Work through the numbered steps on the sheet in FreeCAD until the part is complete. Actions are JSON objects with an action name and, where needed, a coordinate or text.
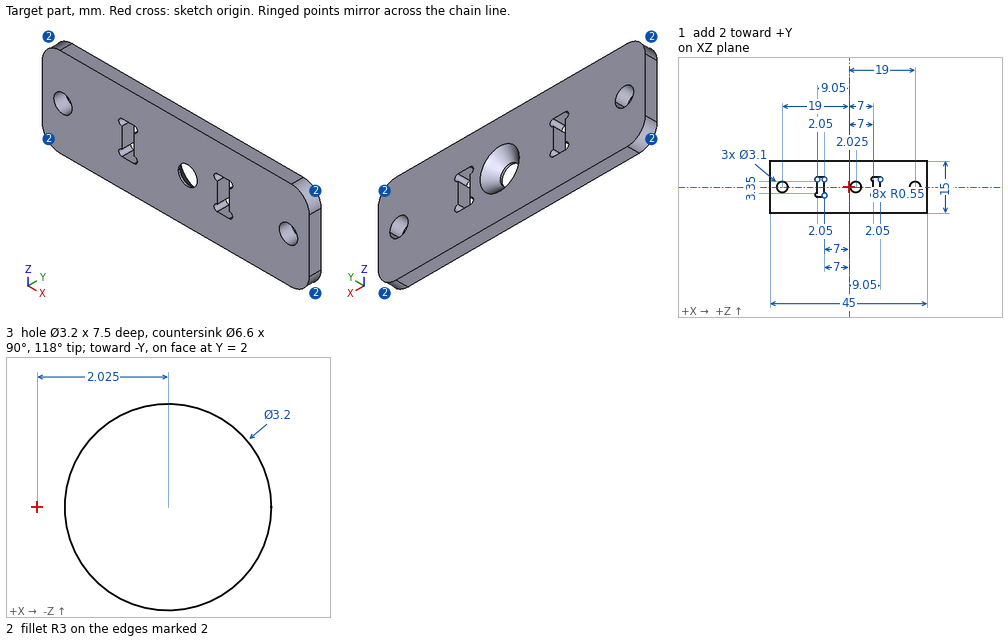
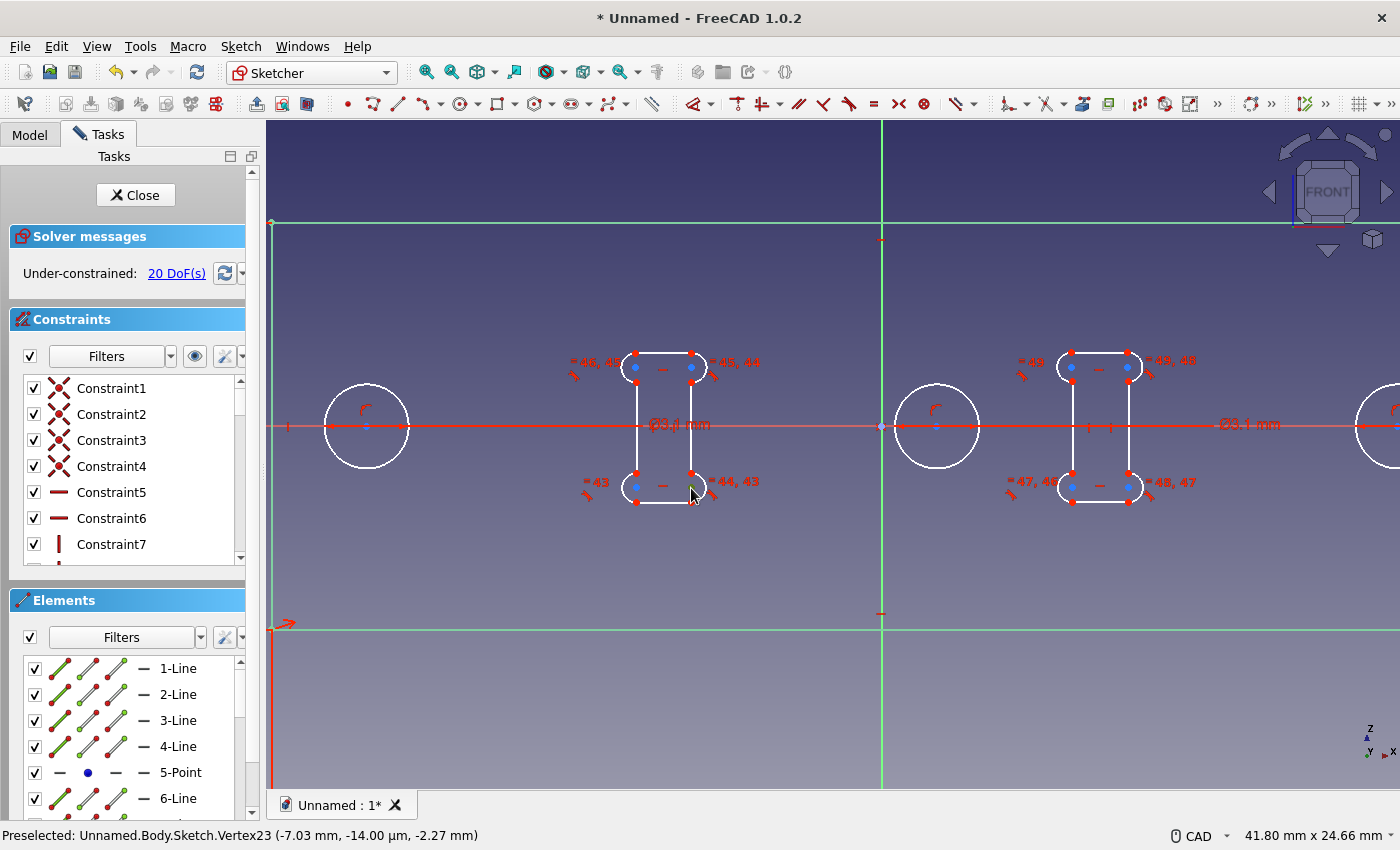
{"action": "left_click", "coordinate": [692, 368]}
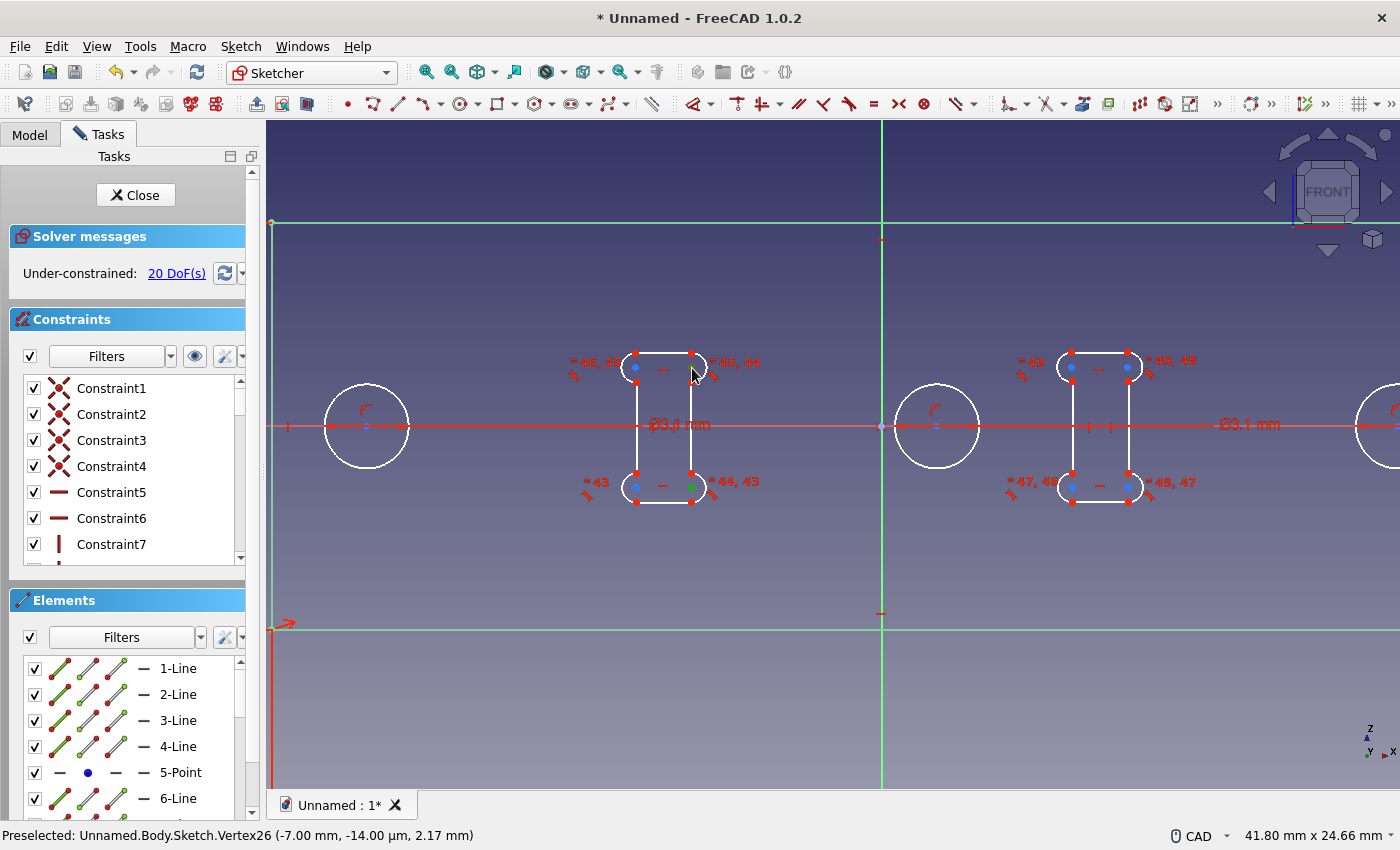
{"action": "left_click", "coordinate": [361, 426]}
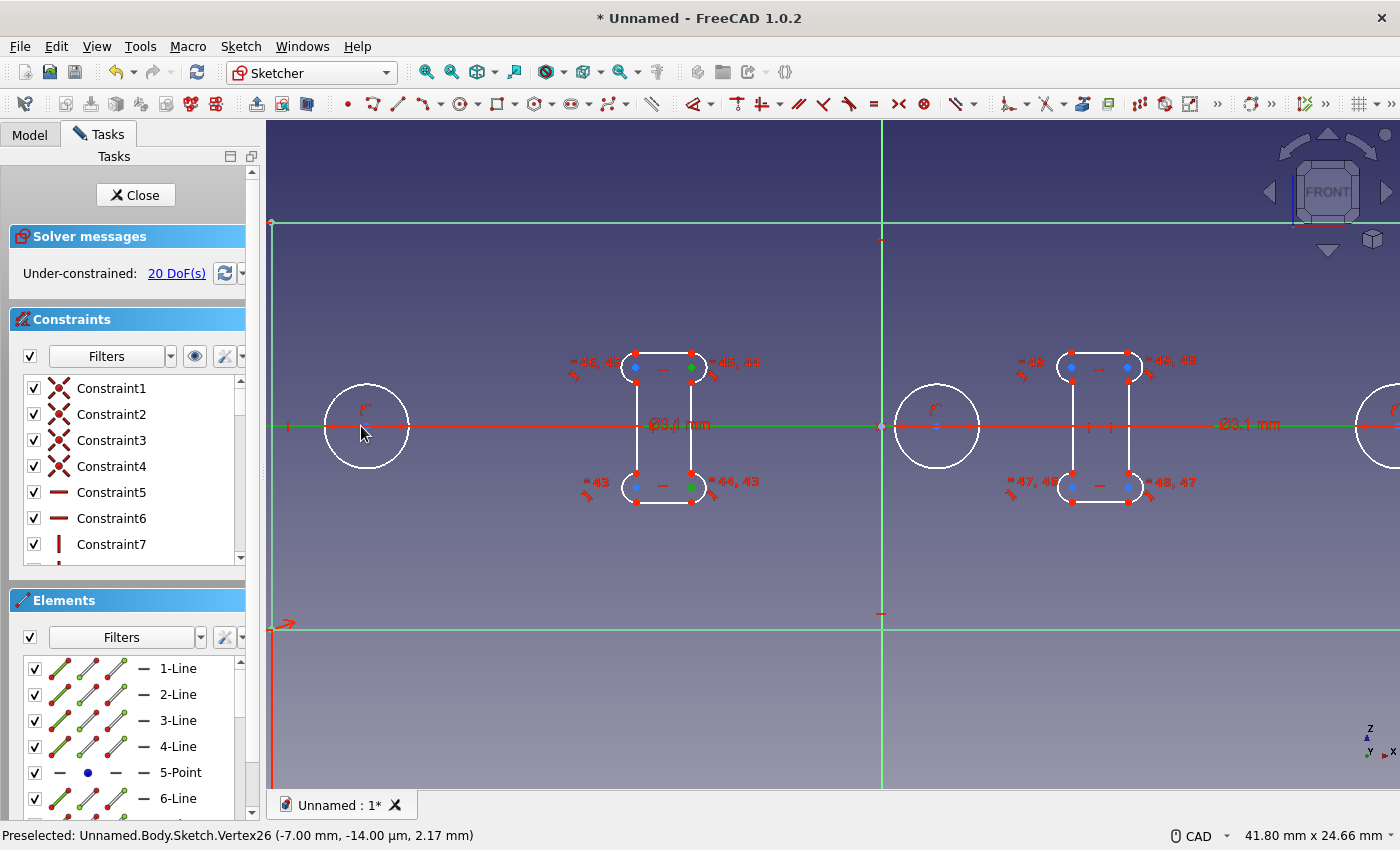
{"action": "left_click", "coordinate": [899, 104]}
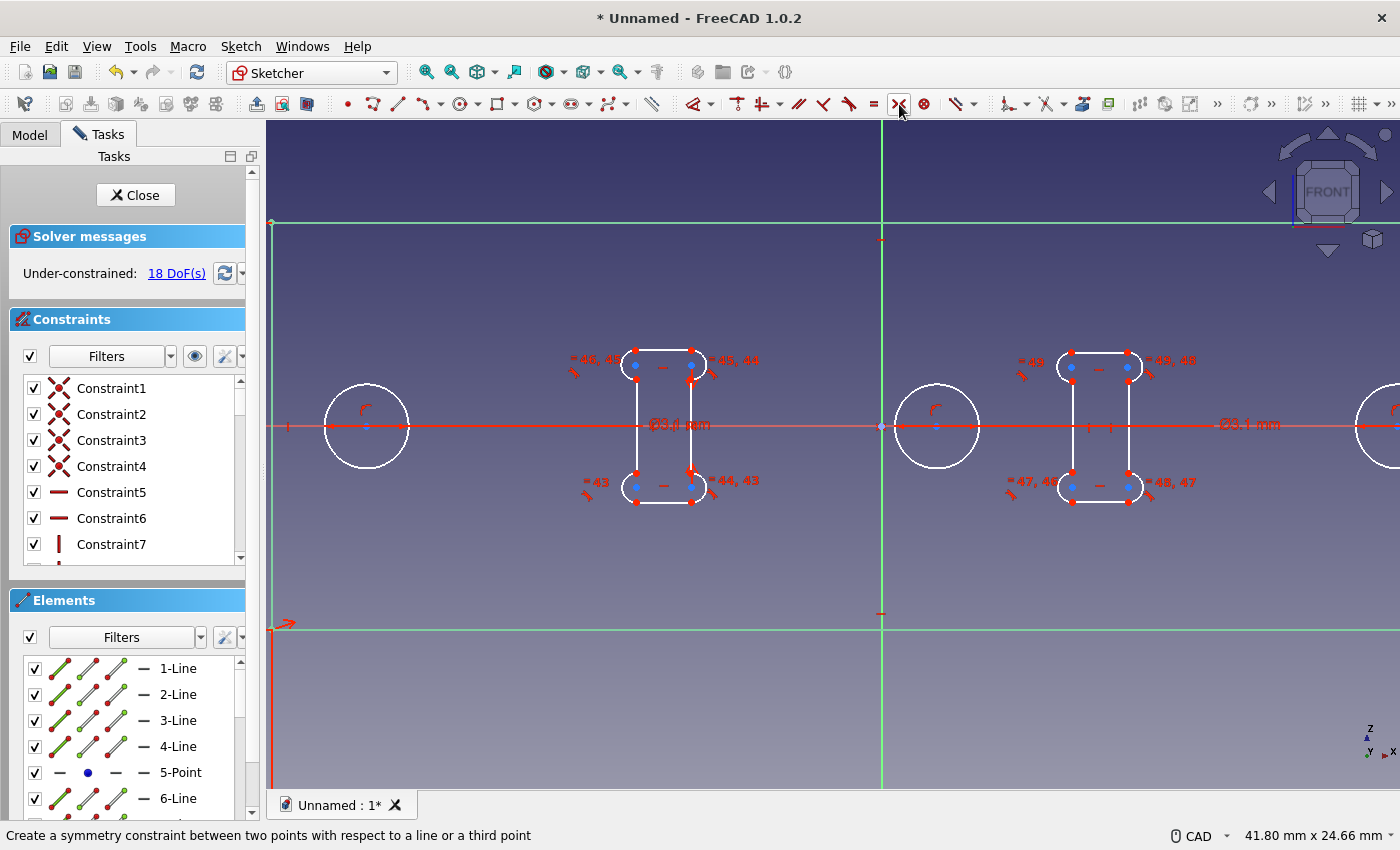
{"action": "left_click", "coordinate": [692, 488]}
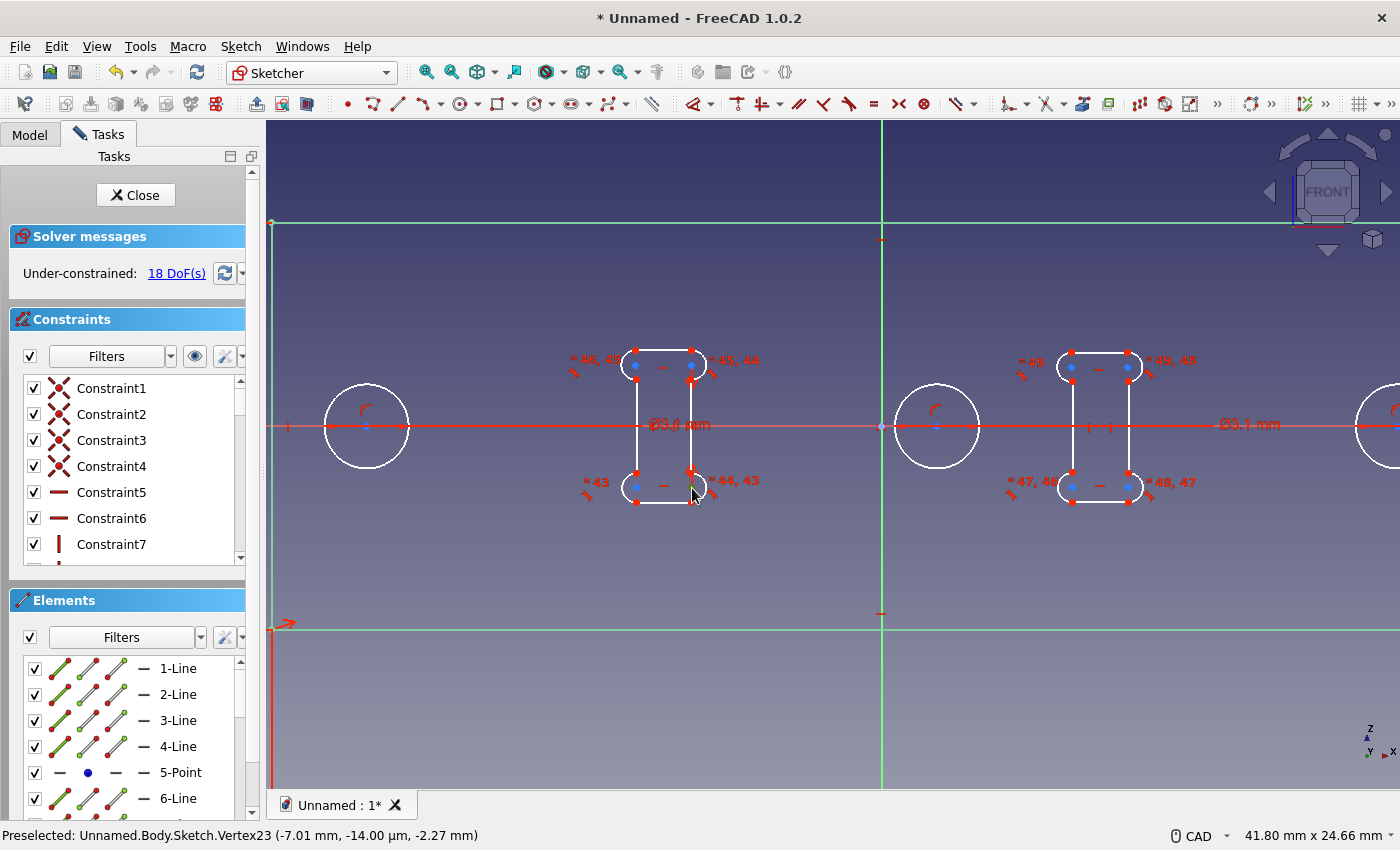
{"action": "left_click", "coordinate": [1072, 488]}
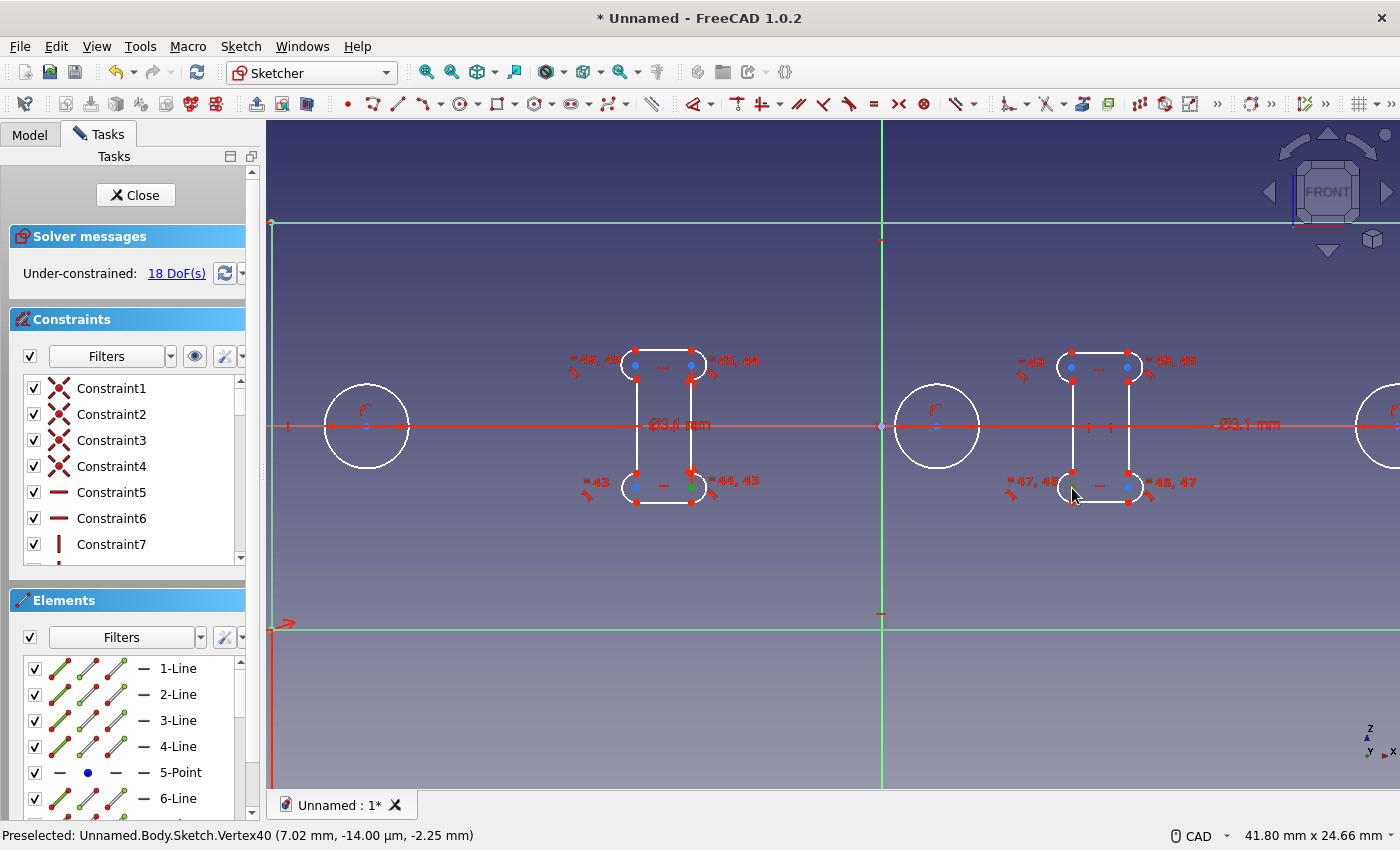
{"action": "left_click", "coordinate": [882, 717]}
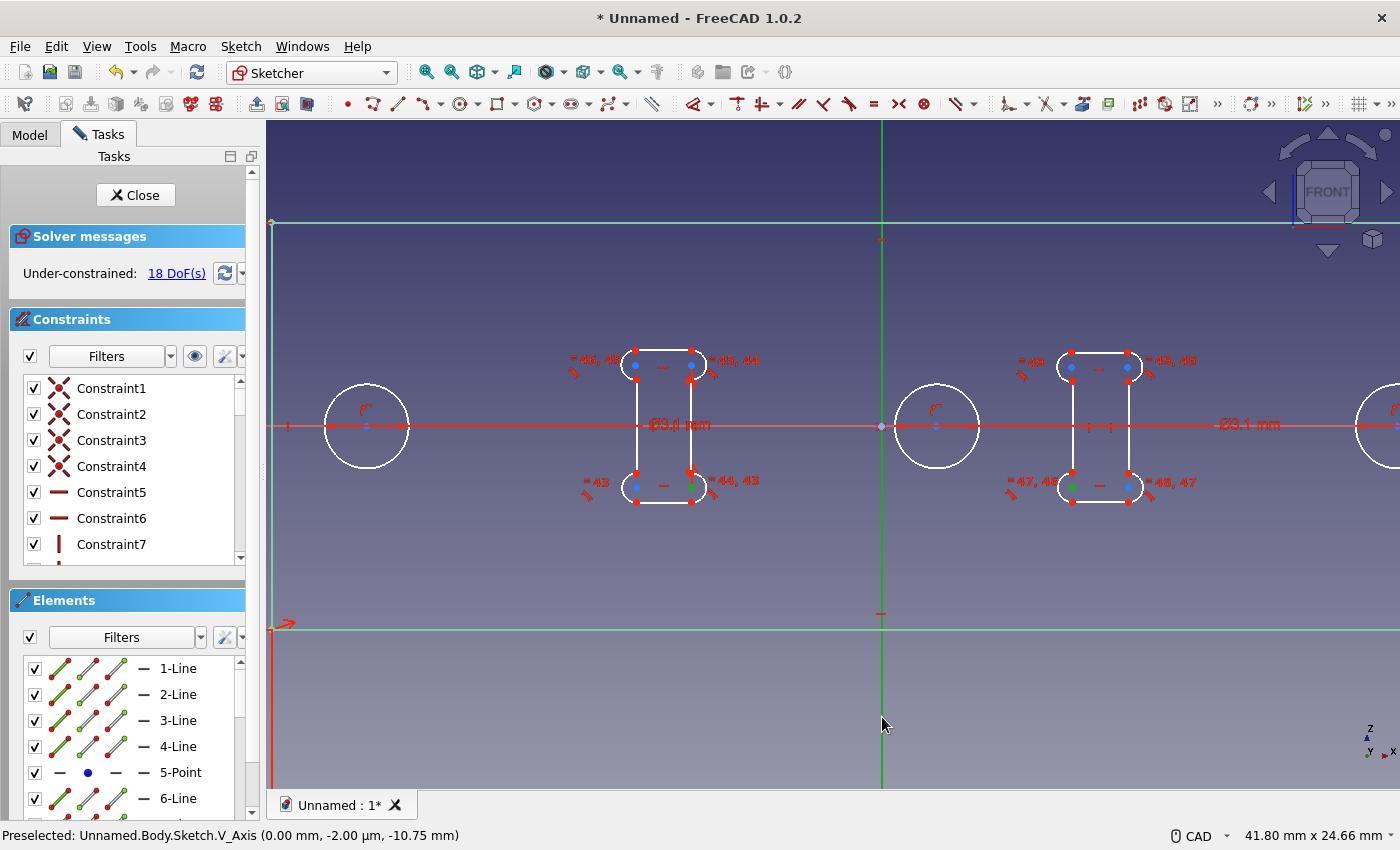
{"action": "left_click", "coordinate": [899, 104]}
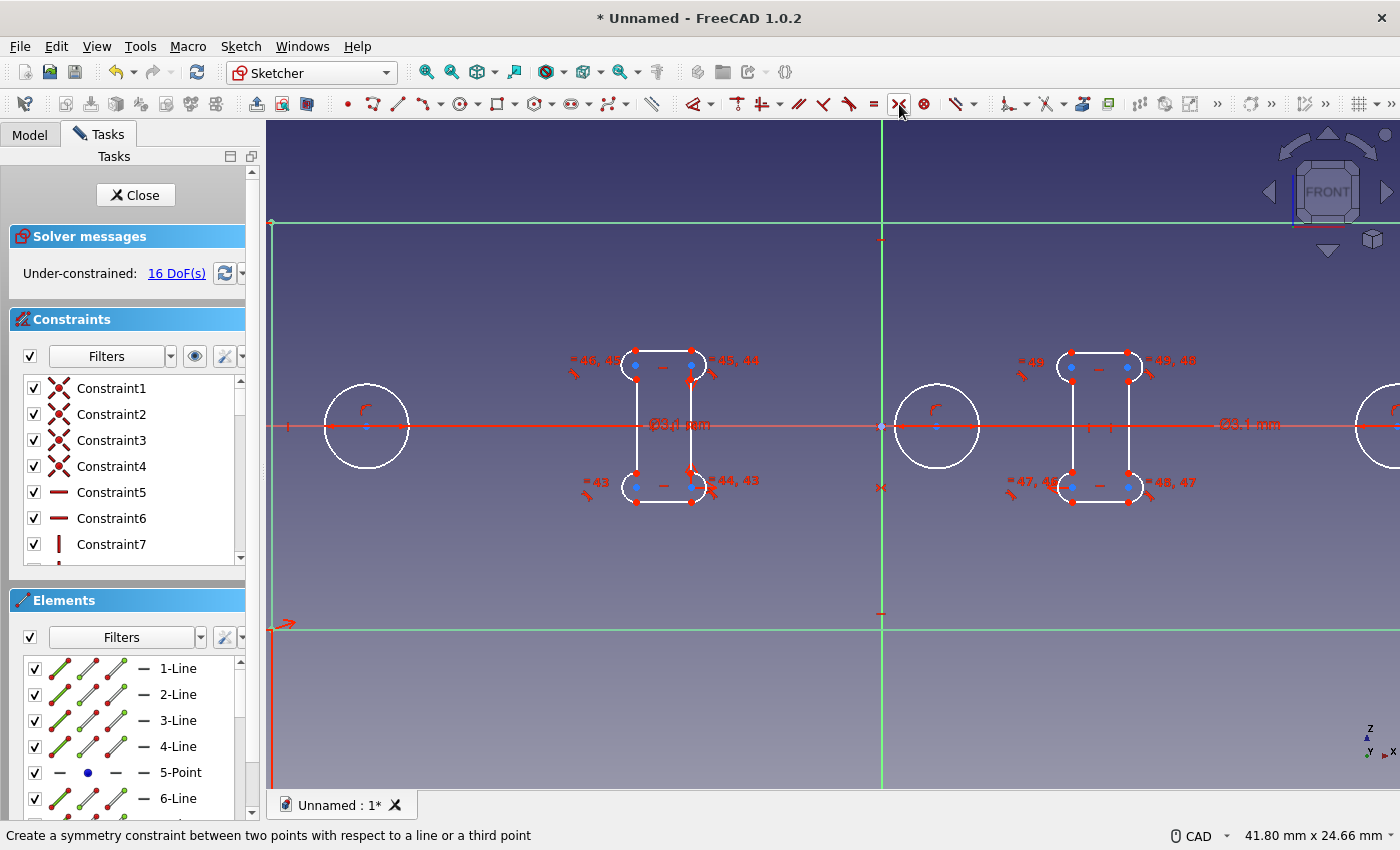
{"action": "left_click", "coordinate": [636, 365]}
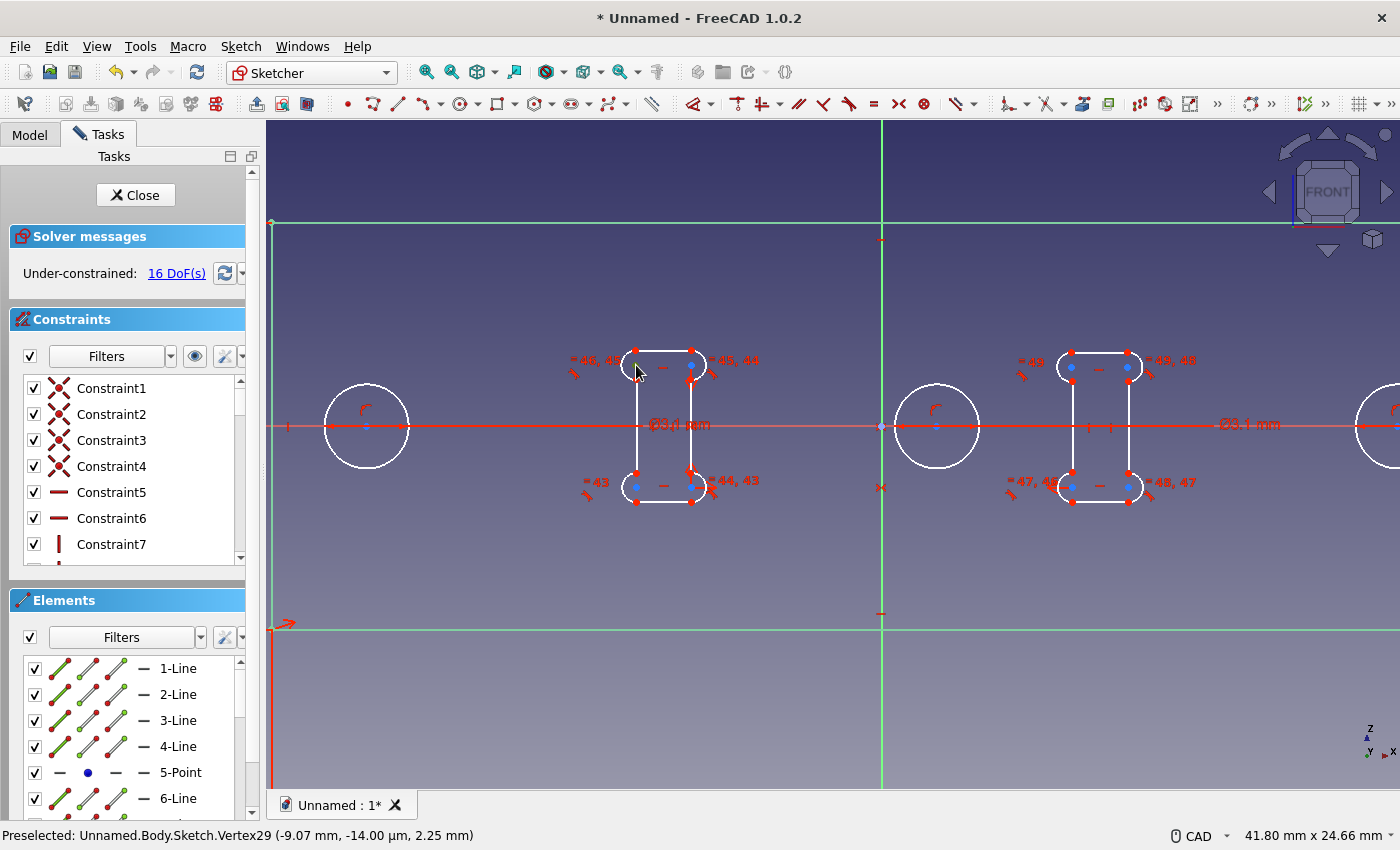
{"action": "left_click", "coordinate": [1128, 367]}